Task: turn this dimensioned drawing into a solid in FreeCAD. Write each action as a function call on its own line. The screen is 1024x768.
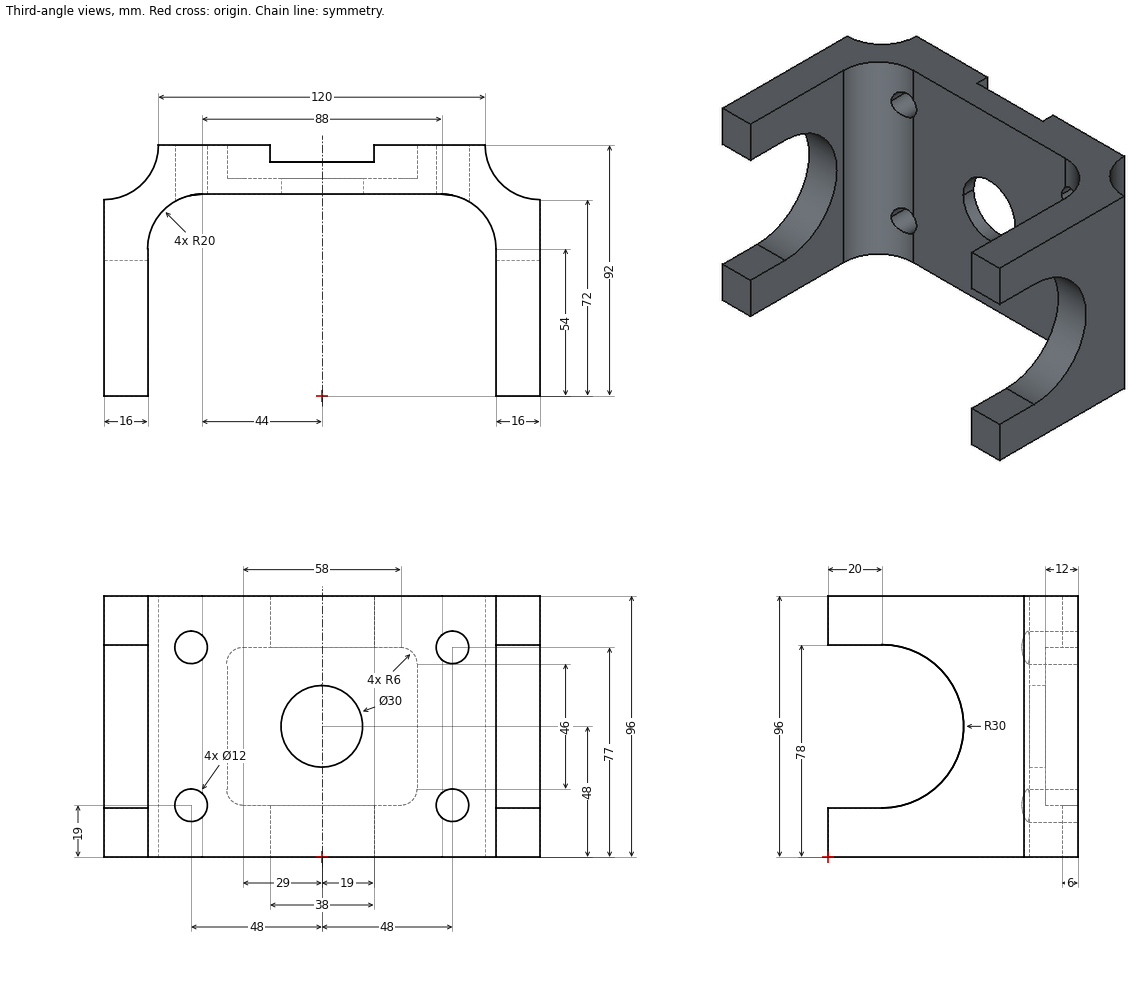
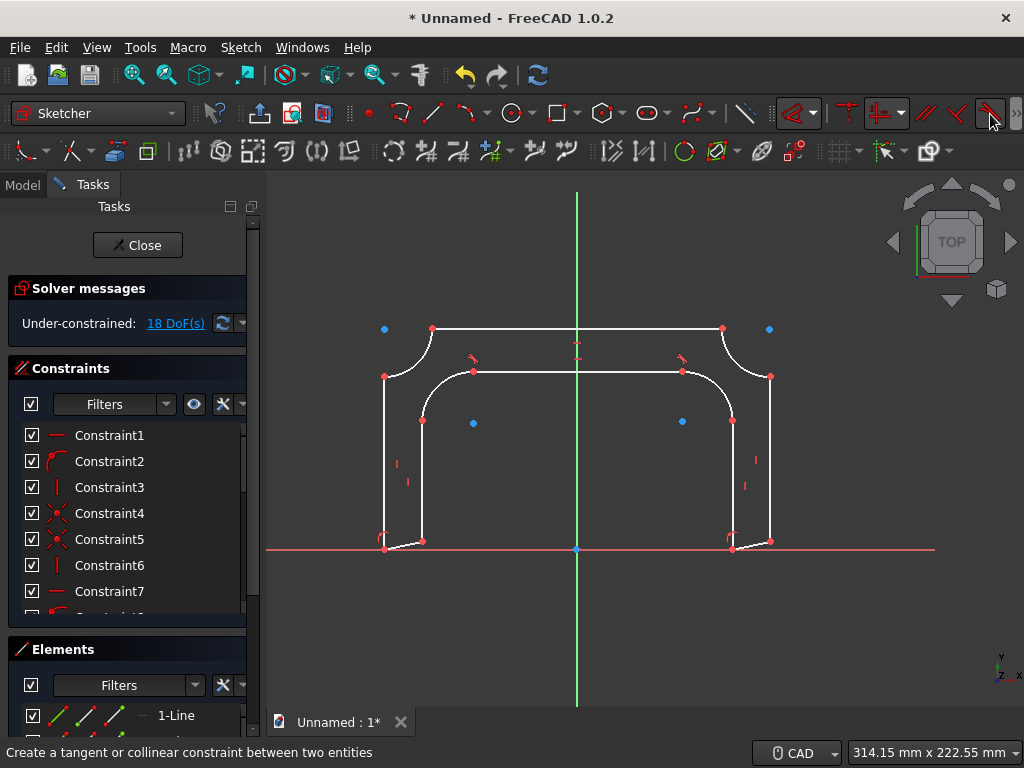
click(733, 460)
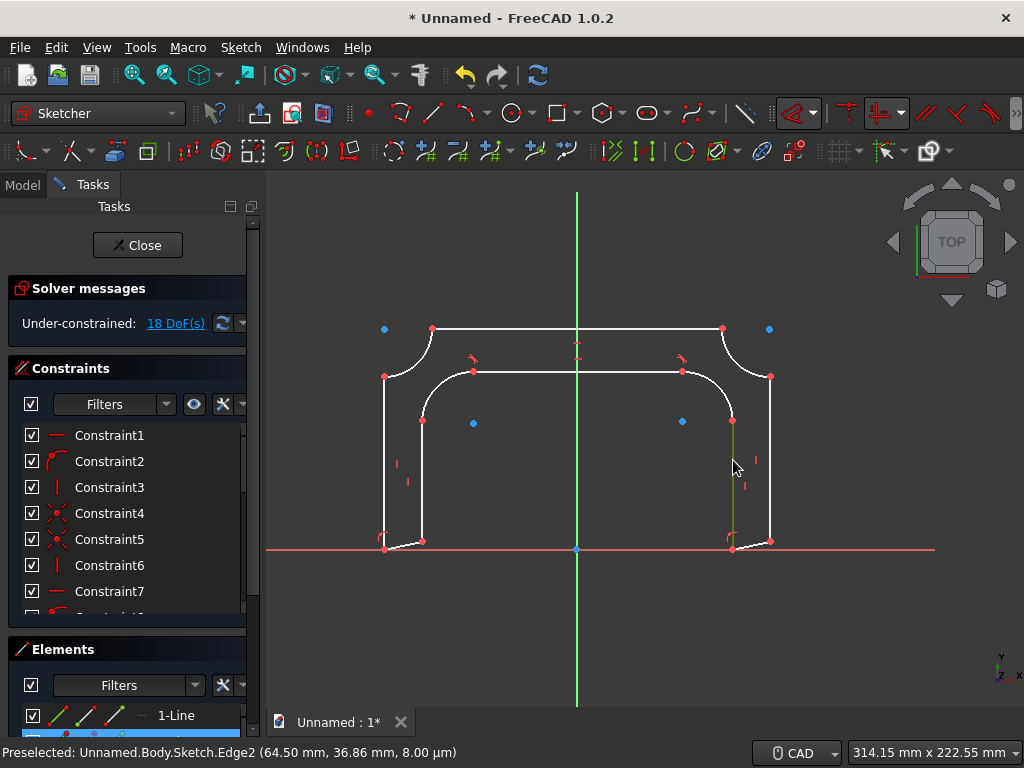
click(727, 399)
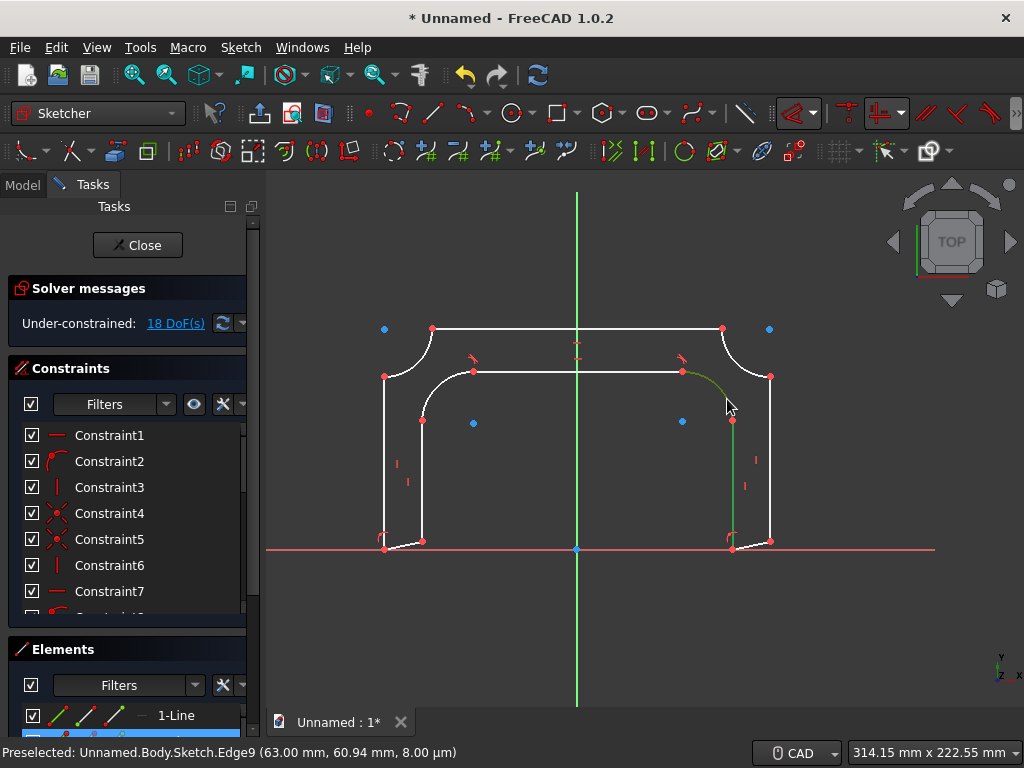
click(990, 114)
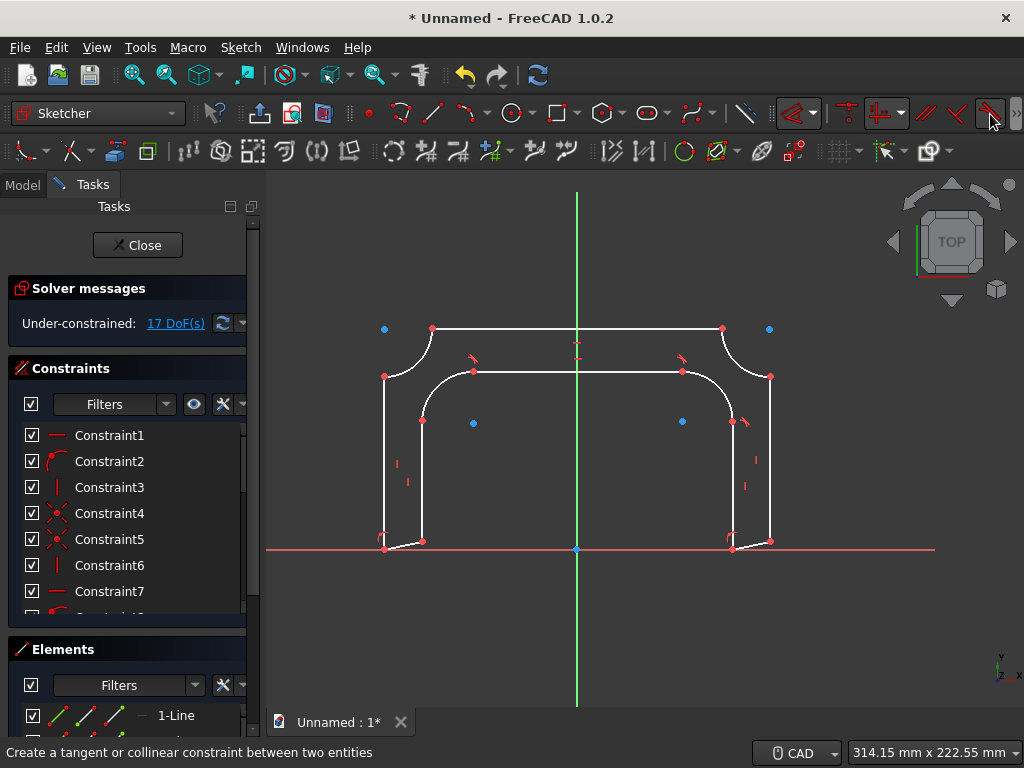
click(422, 506)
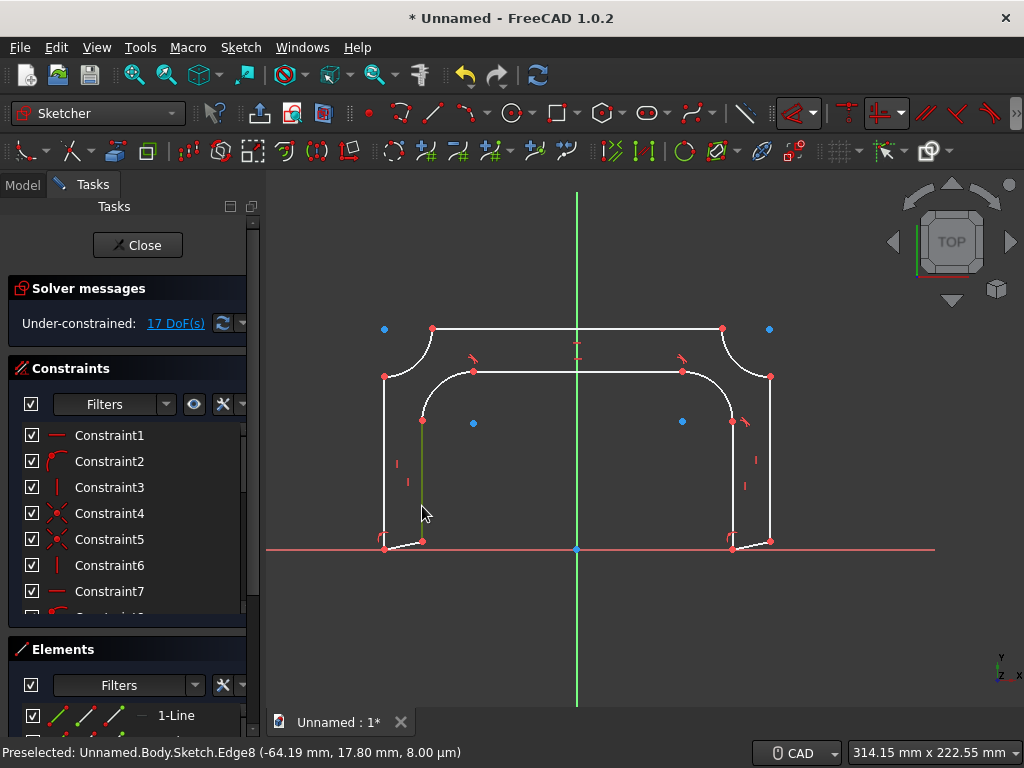
click(451, 377)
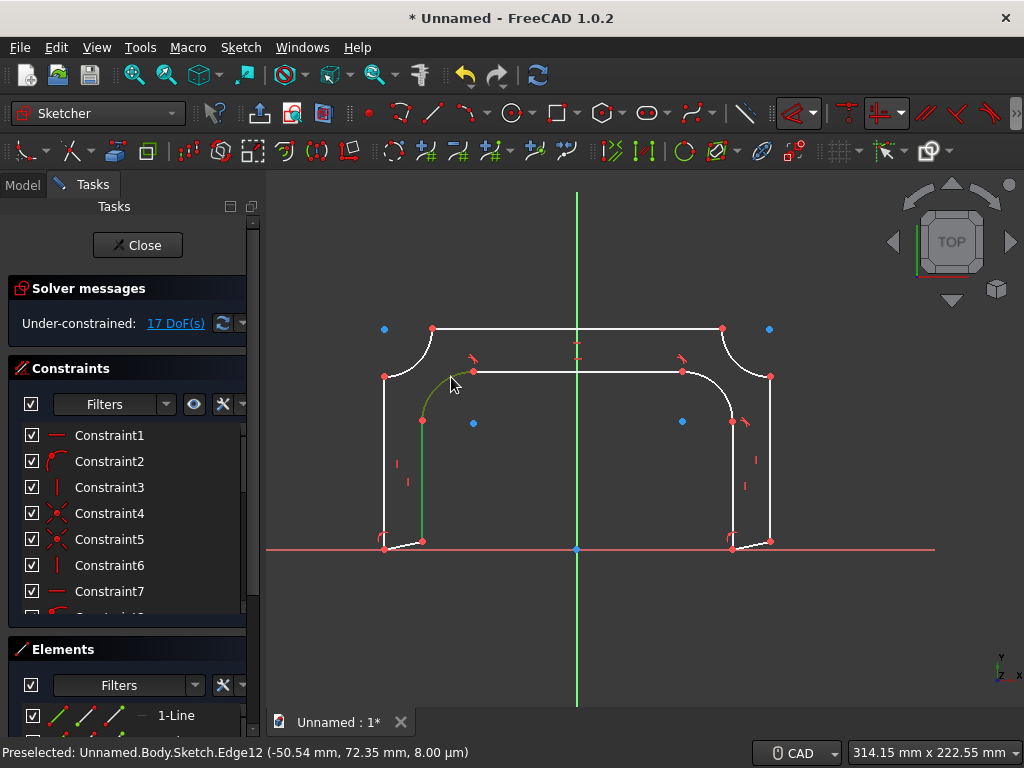
click(990, 114)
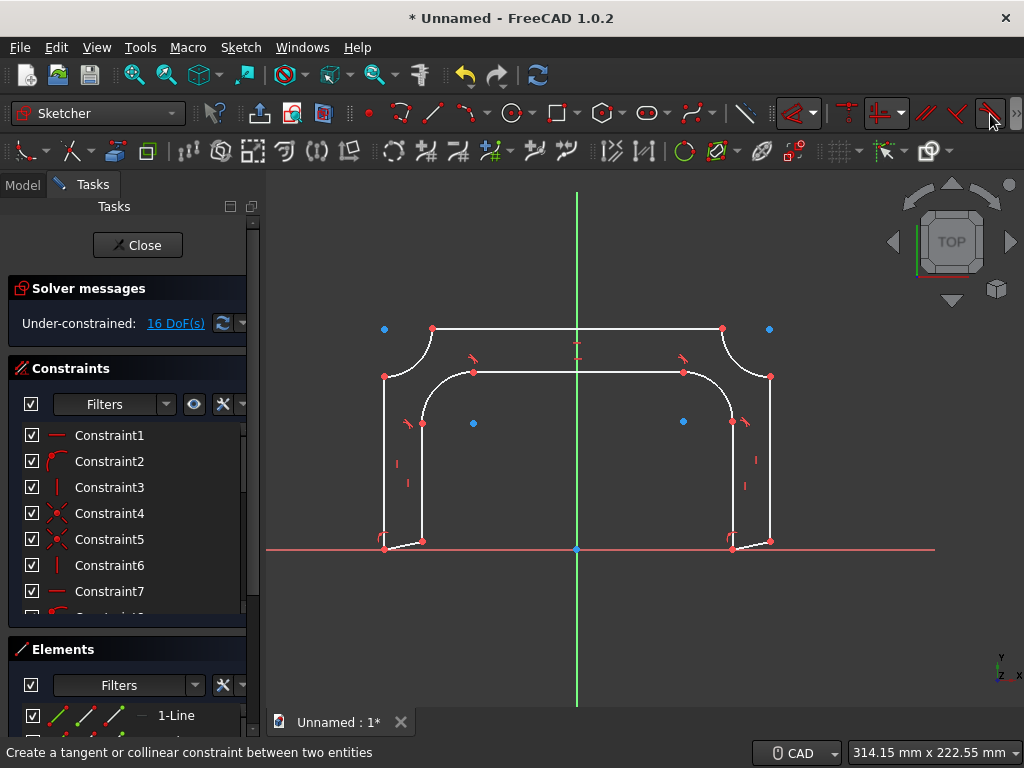
scroll(744, 548, up, 2)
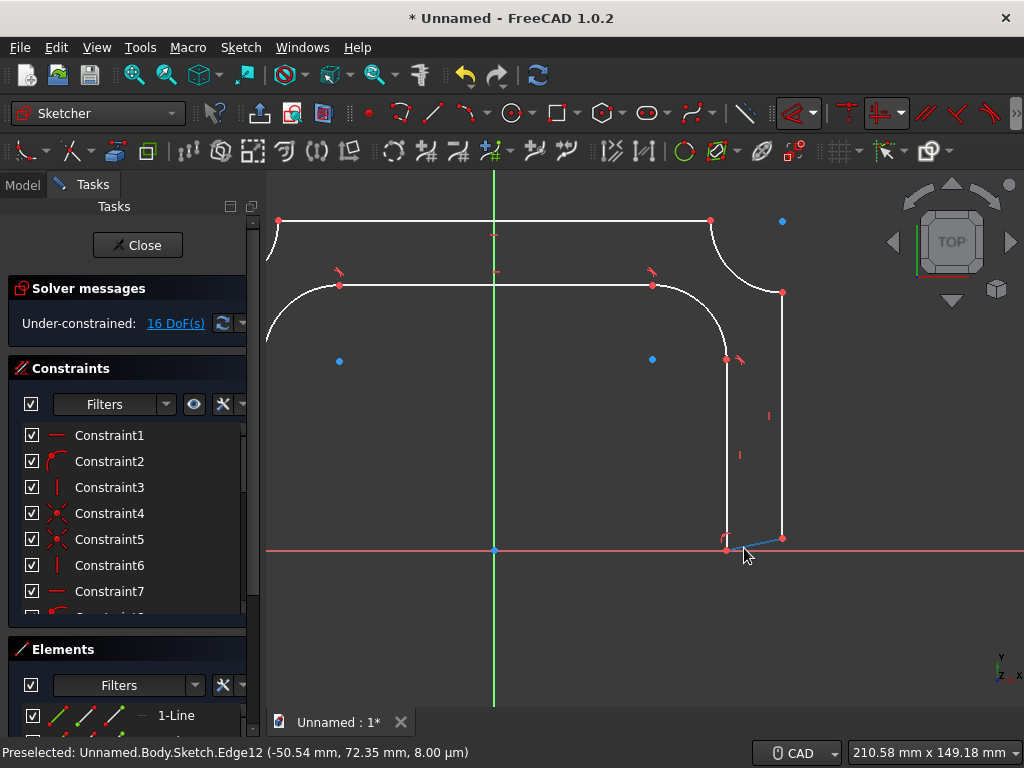
click(743, 547)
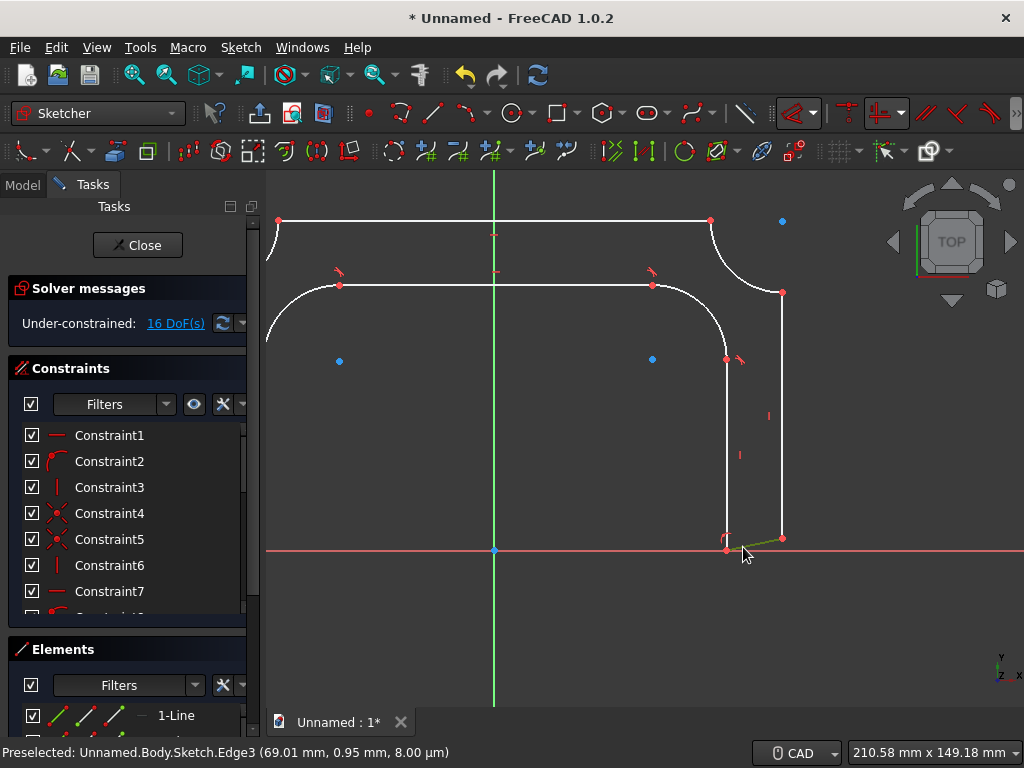
key(h)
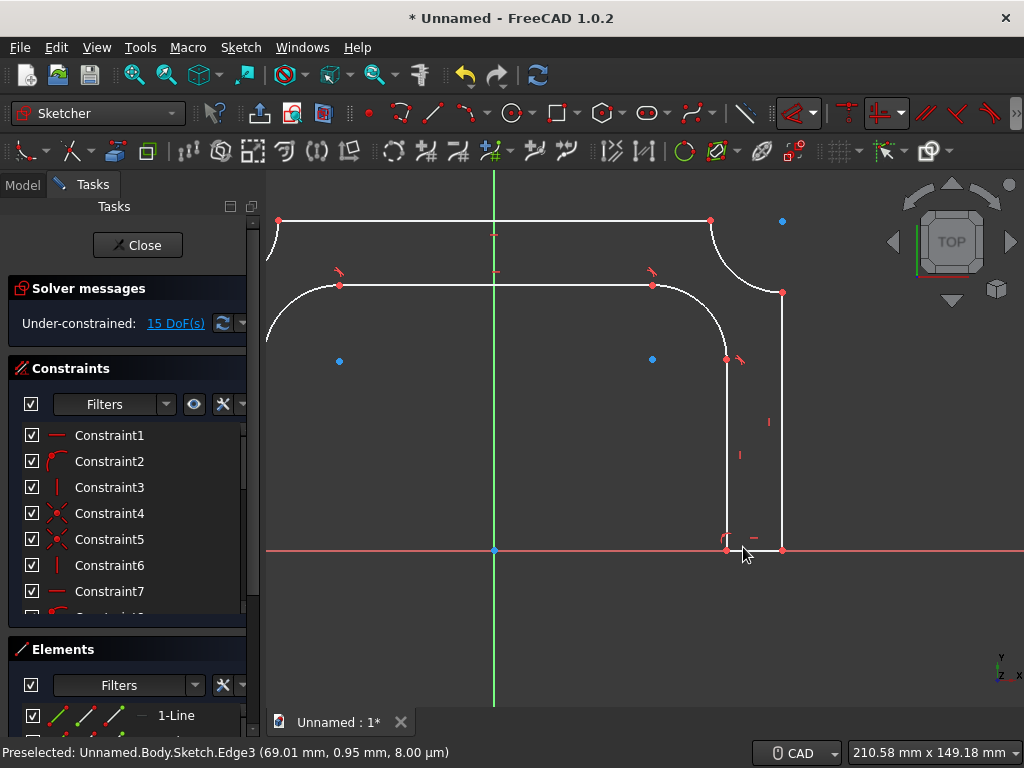
scroll(743, 547, down, 2)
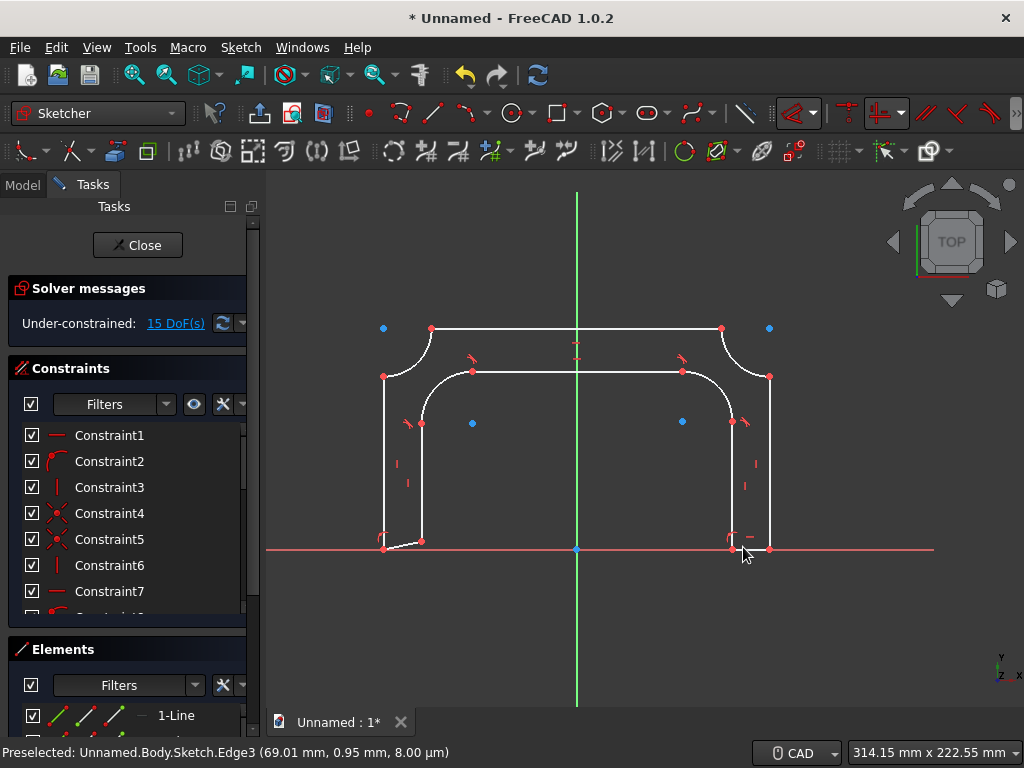
click(395, 547)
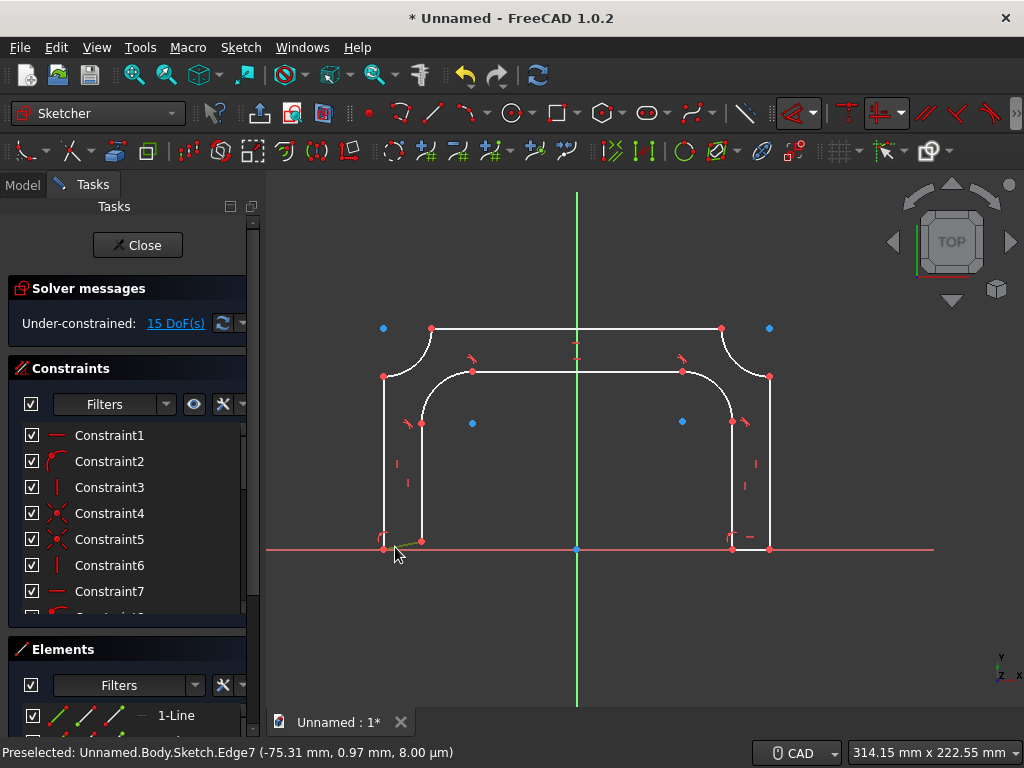
click(904, 114)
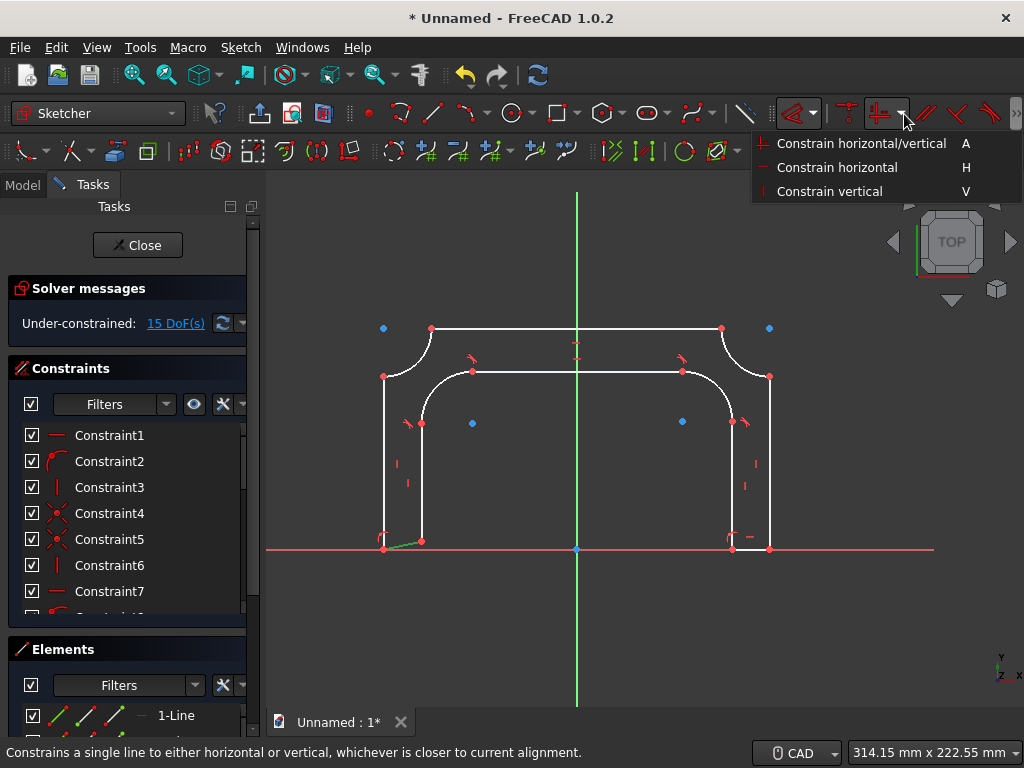
click(887, 167)